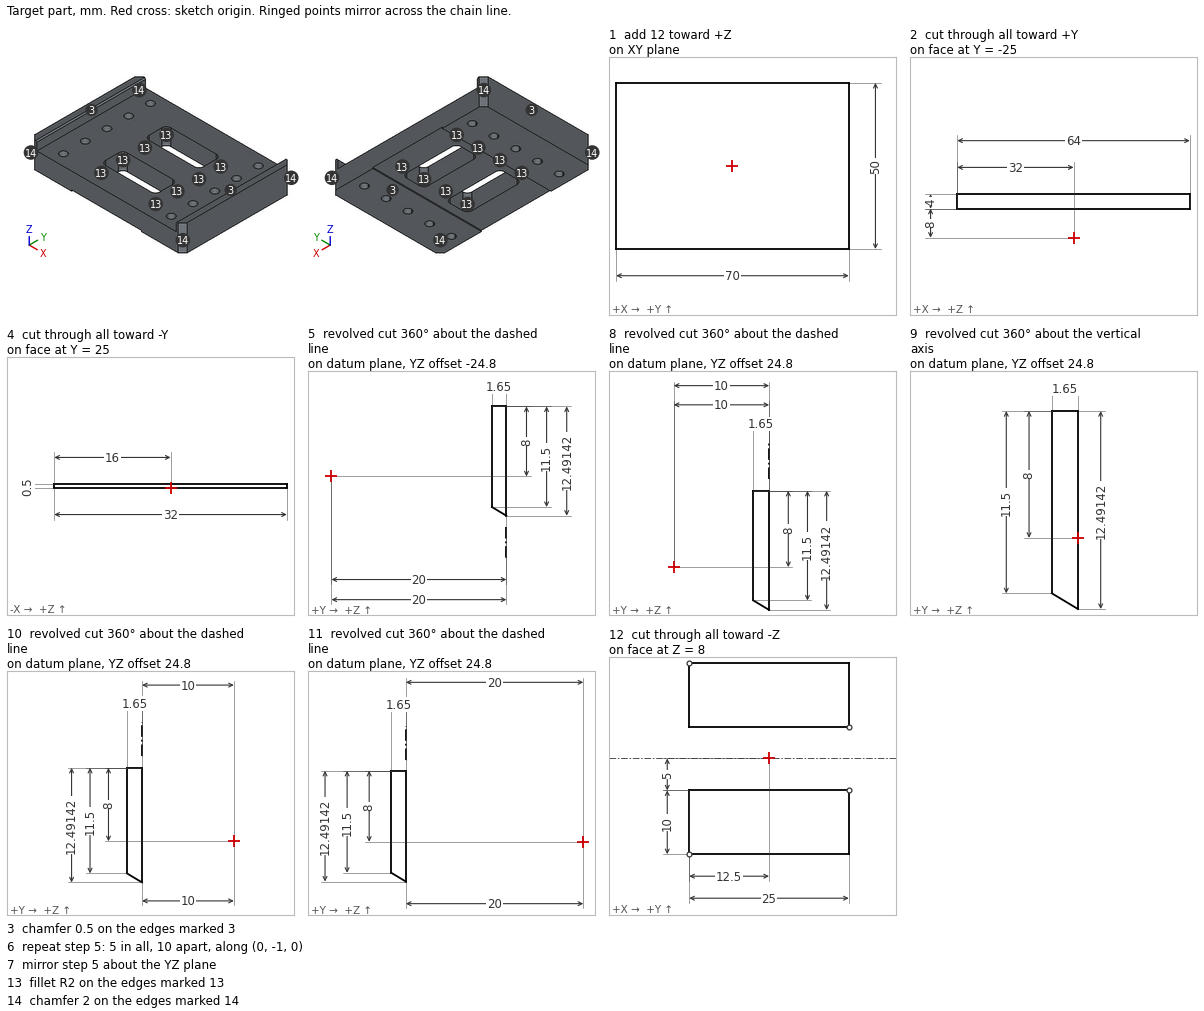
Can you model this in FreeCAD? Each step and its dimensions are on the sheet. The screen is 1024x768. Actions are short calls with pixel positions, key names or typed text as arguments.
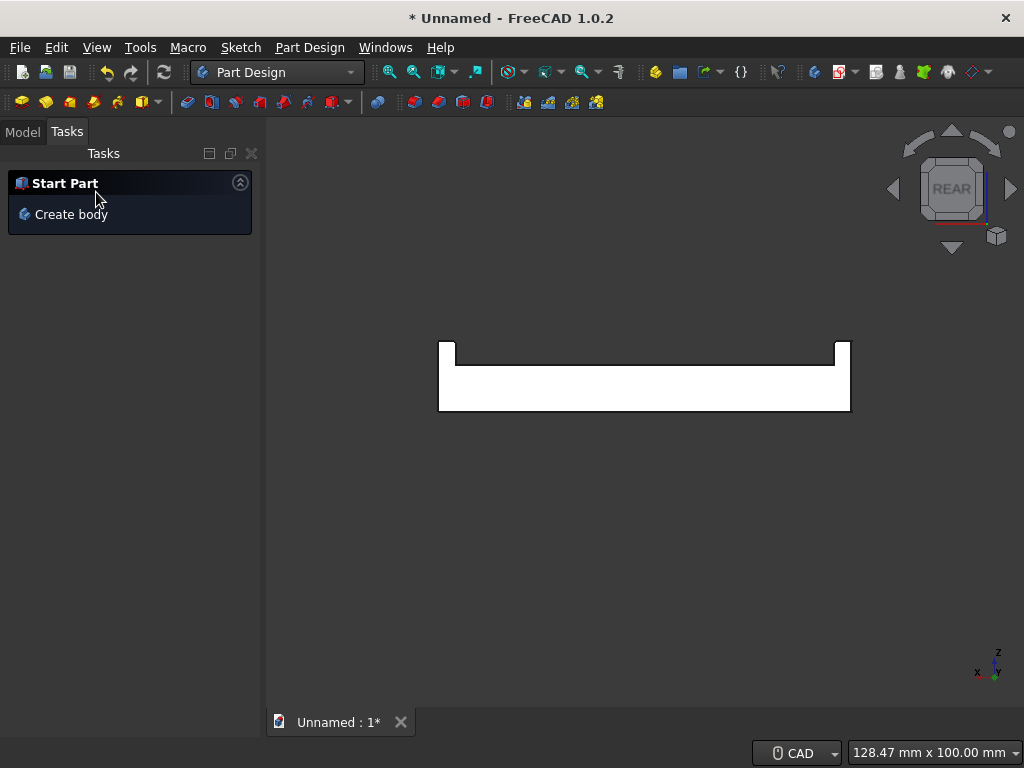
click(468, 386)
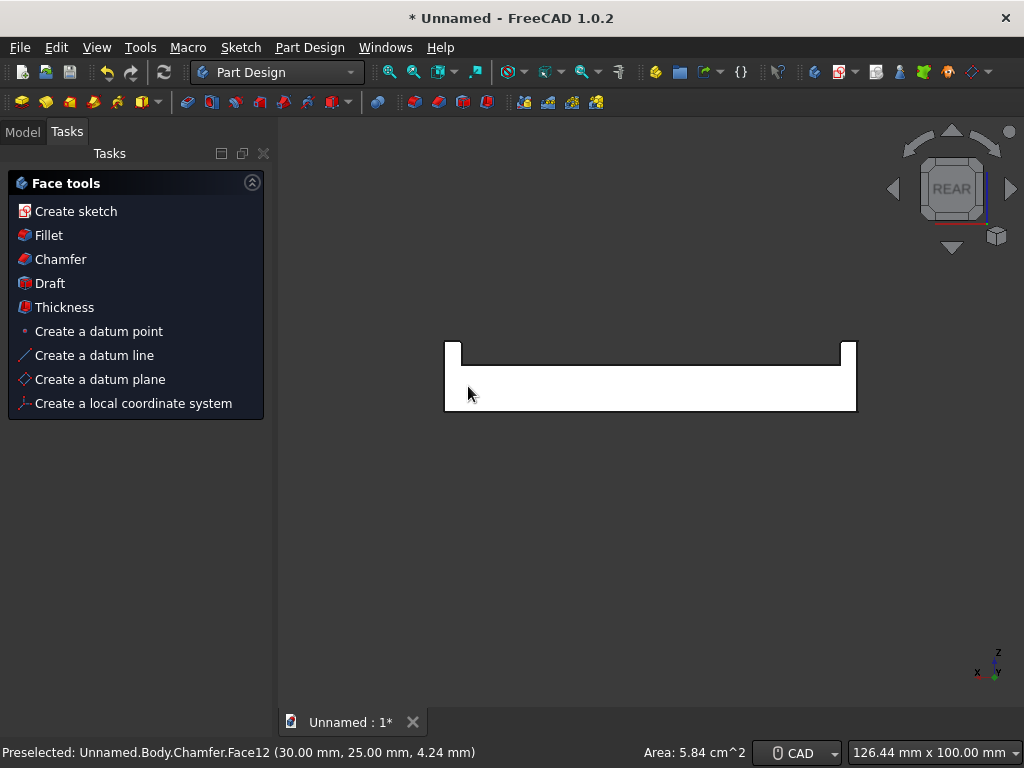
click(840, 72)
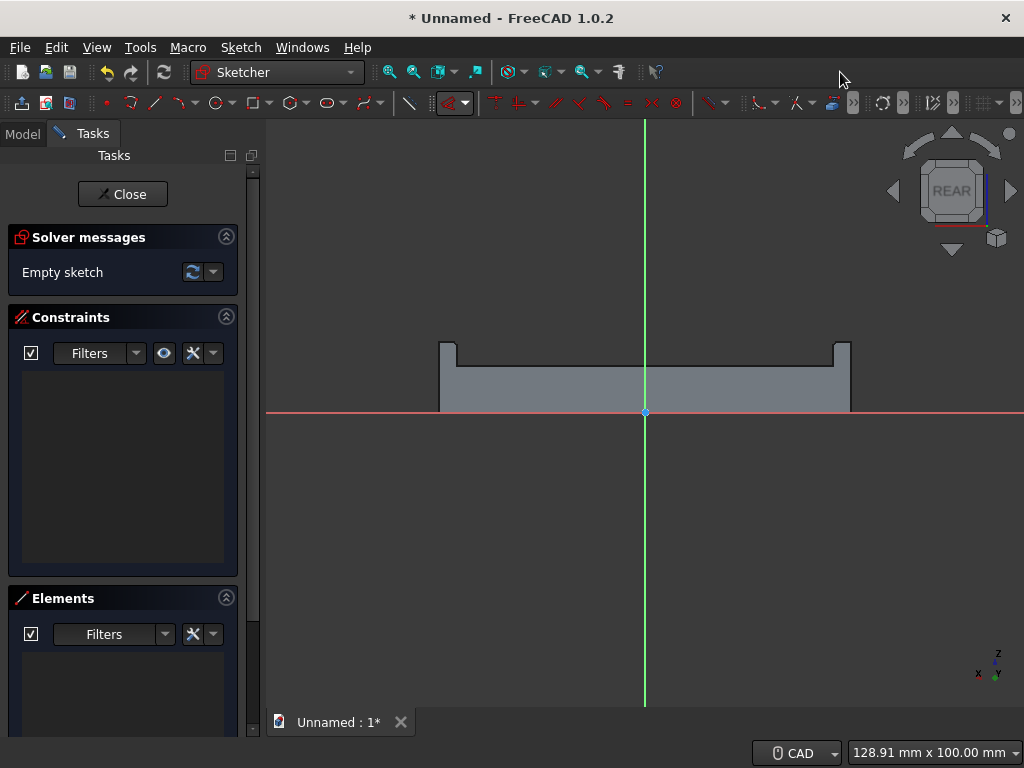
scroll(701, 410, up, 4)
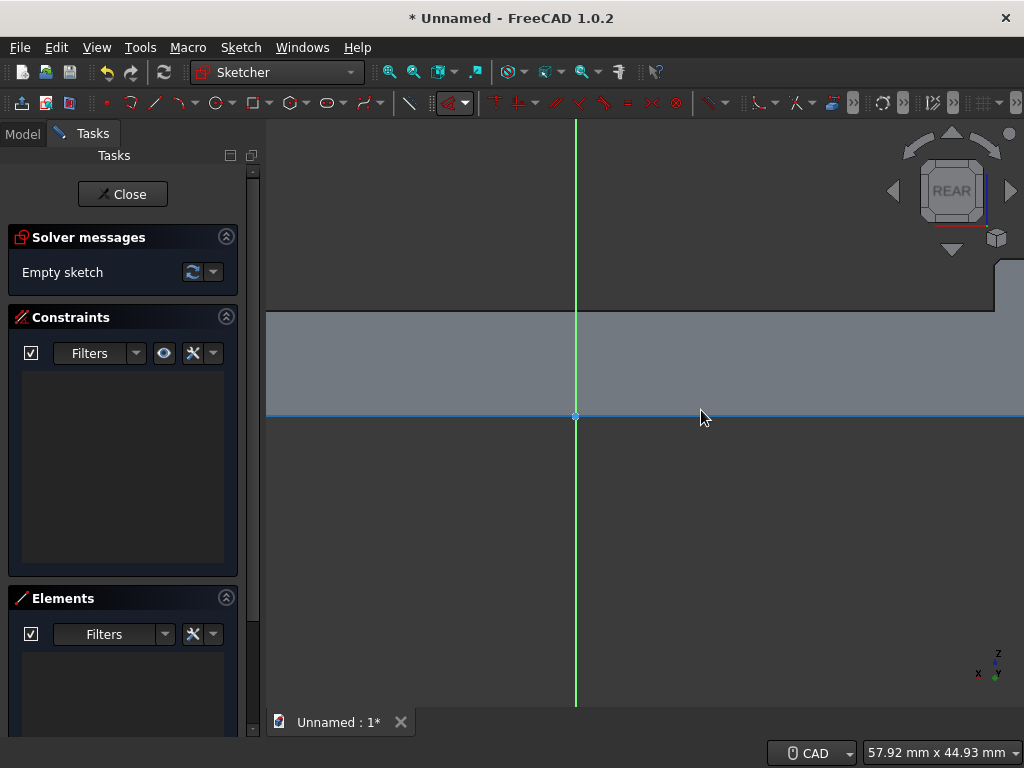
key(g)
key(r)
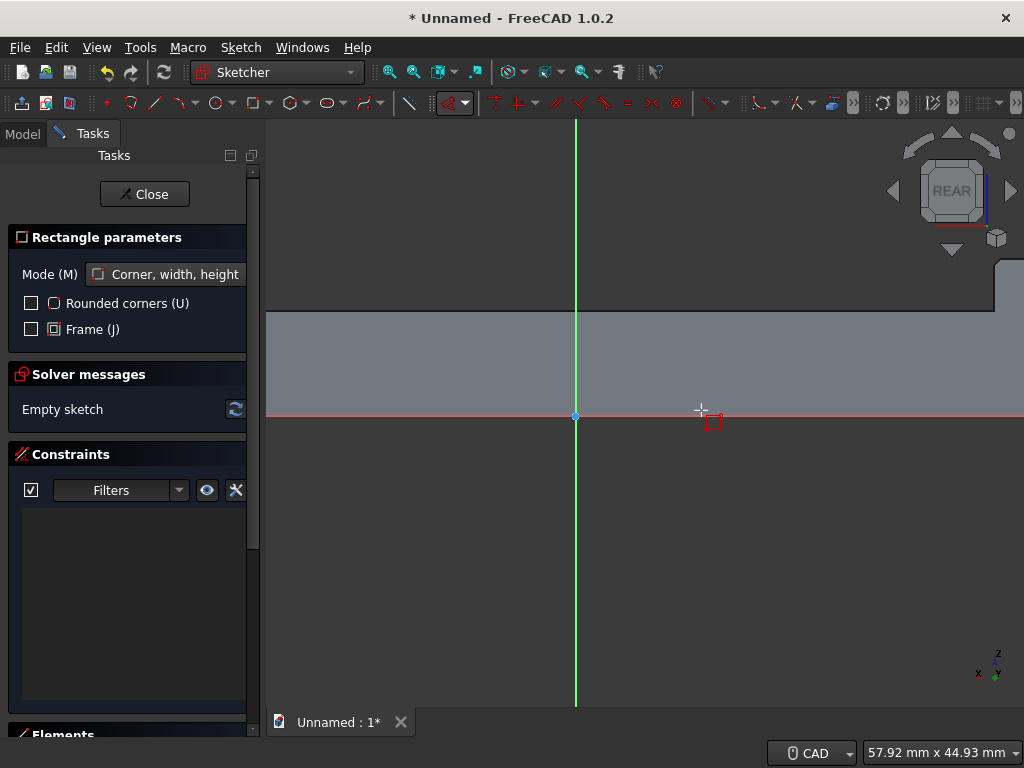
scroll(366, 410, up, 5)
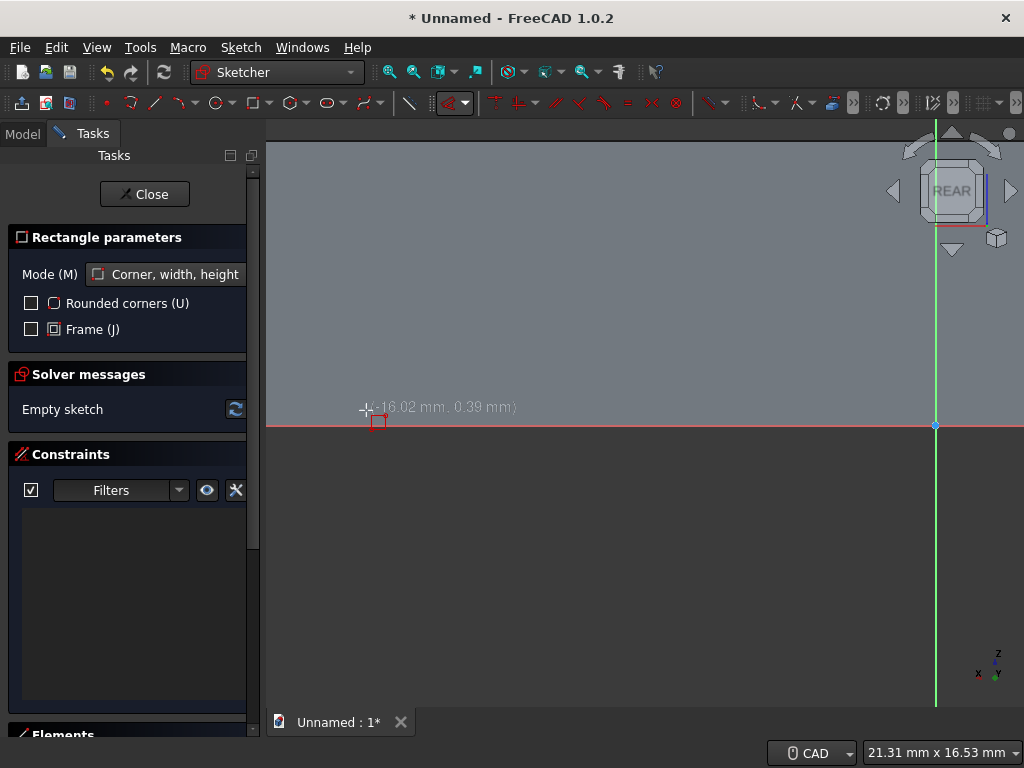
click(367, 408)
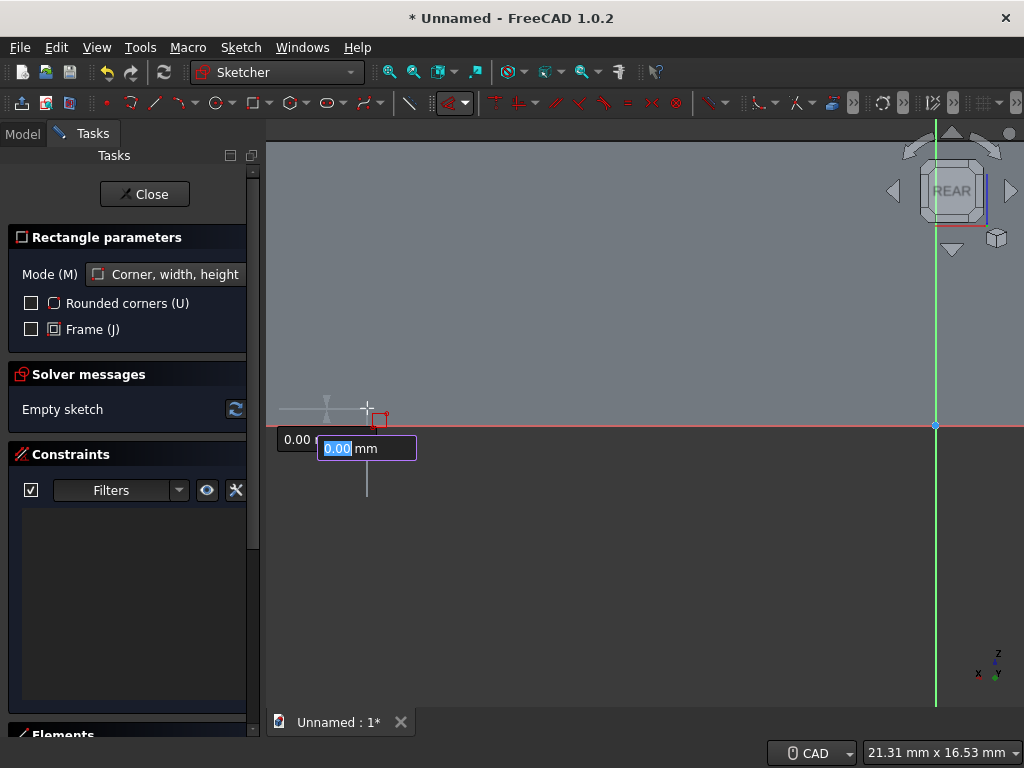
scroll(367, 411, down, 5)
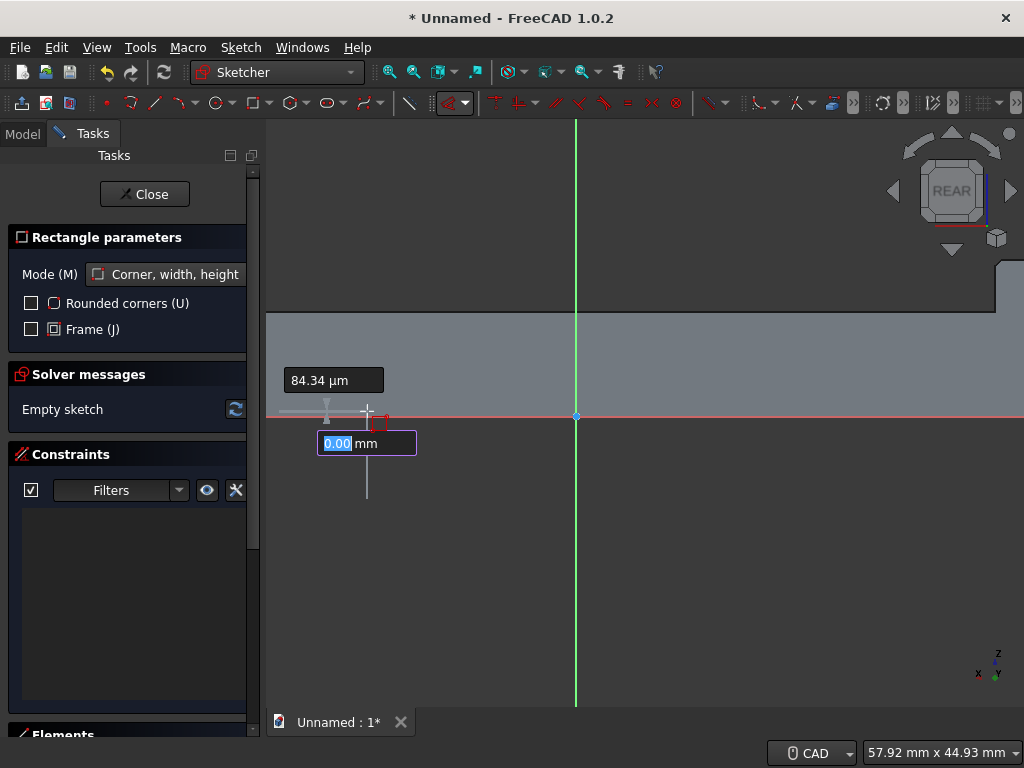
click(786, 417)
key(Escape)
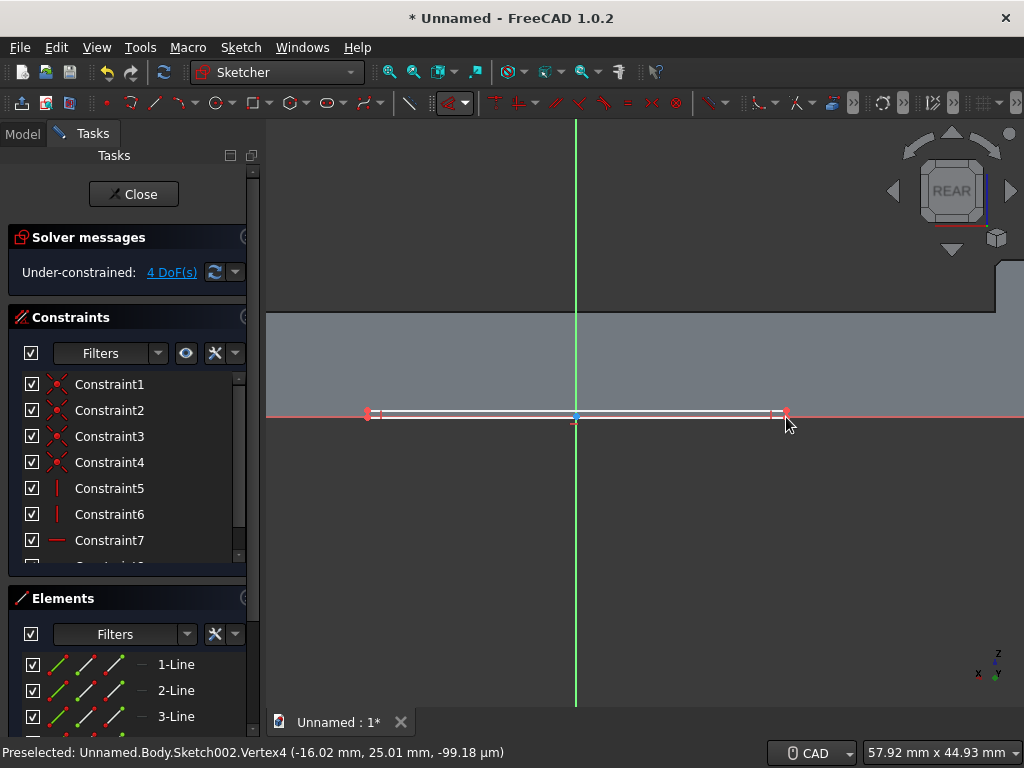
scroll(367, 418, up, 3)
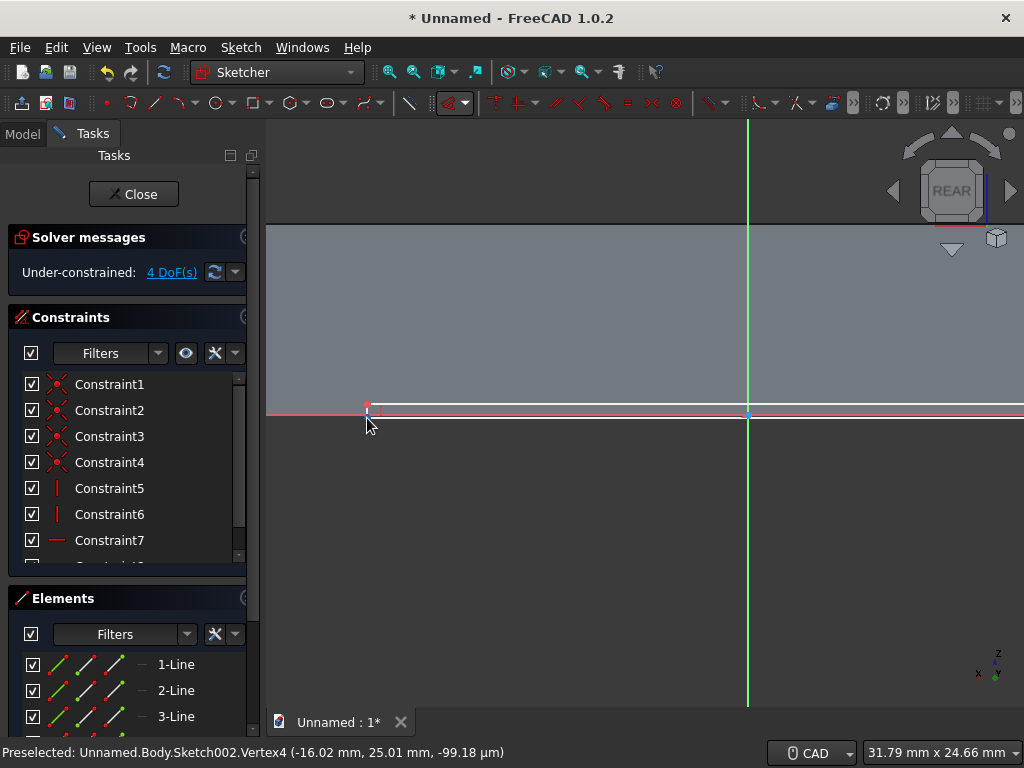
click(367, 418)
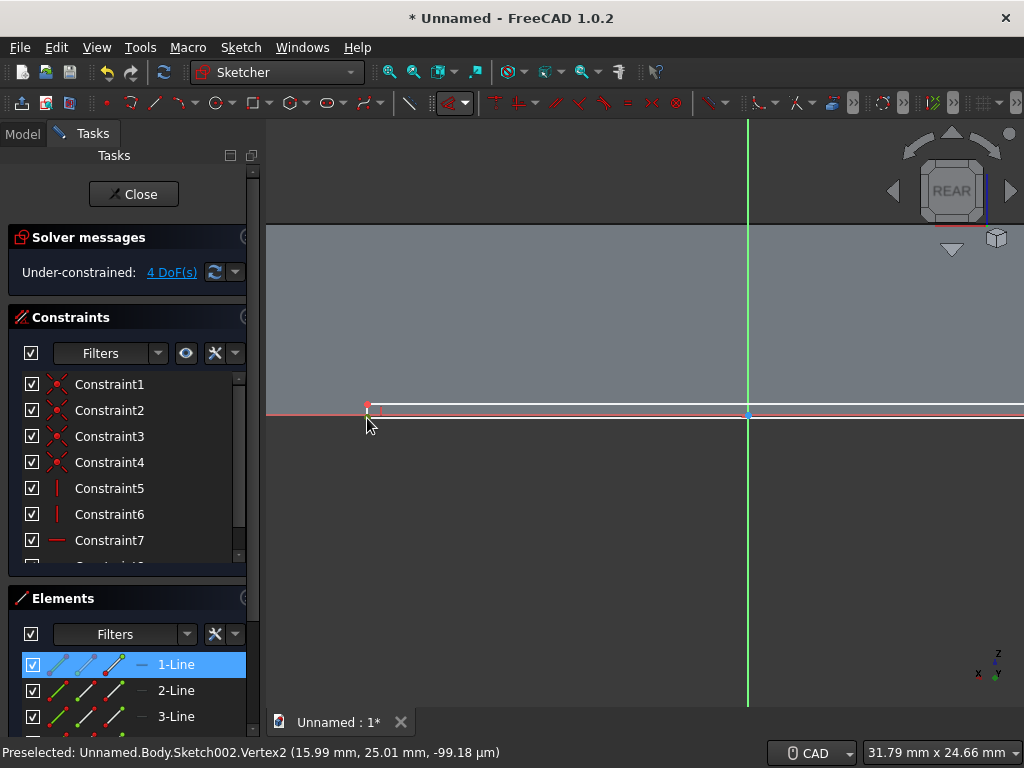
click(334, 415)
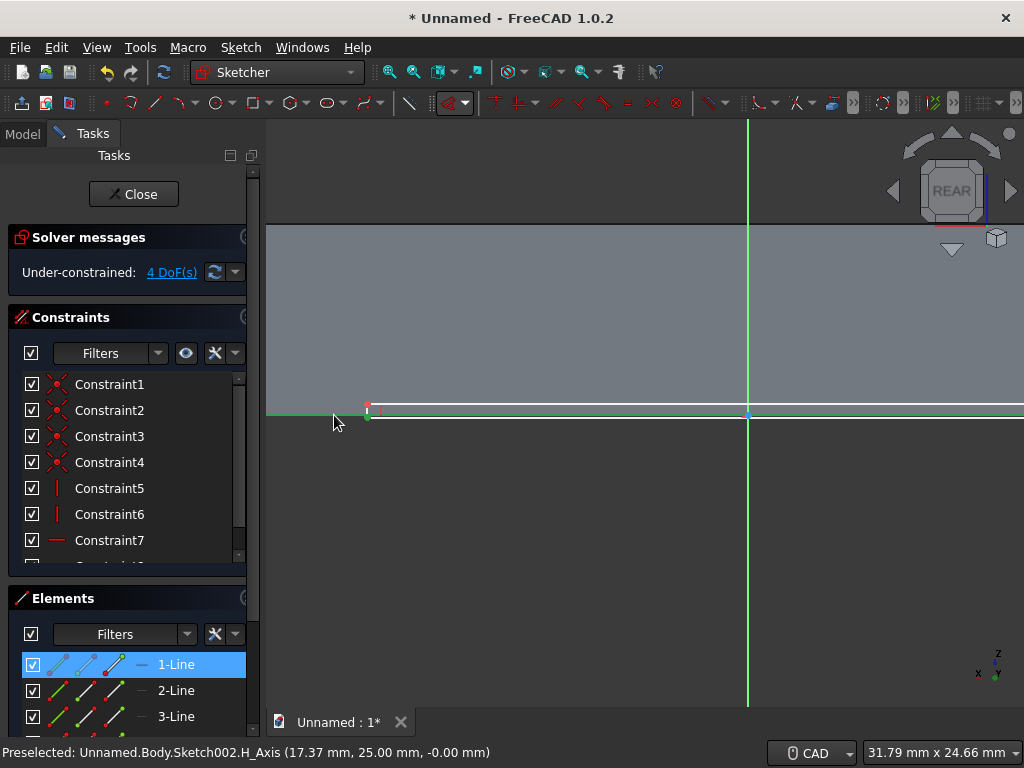
key(c)